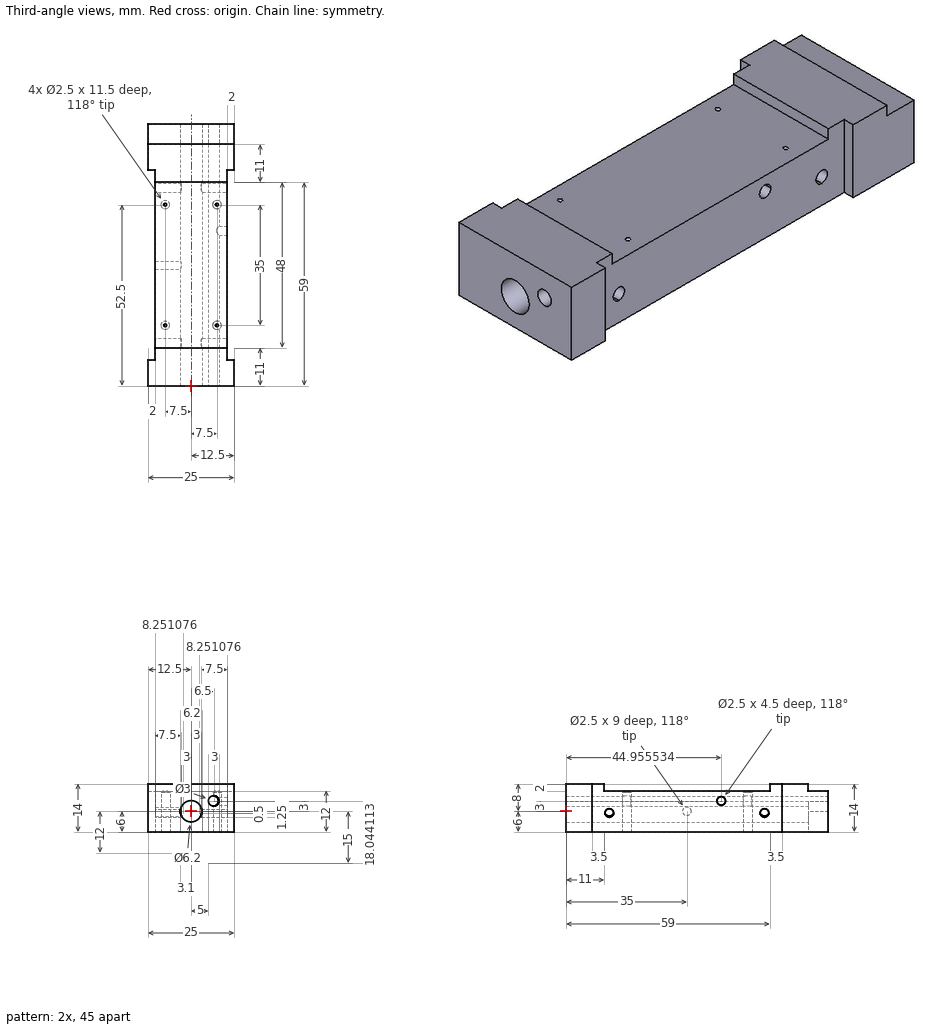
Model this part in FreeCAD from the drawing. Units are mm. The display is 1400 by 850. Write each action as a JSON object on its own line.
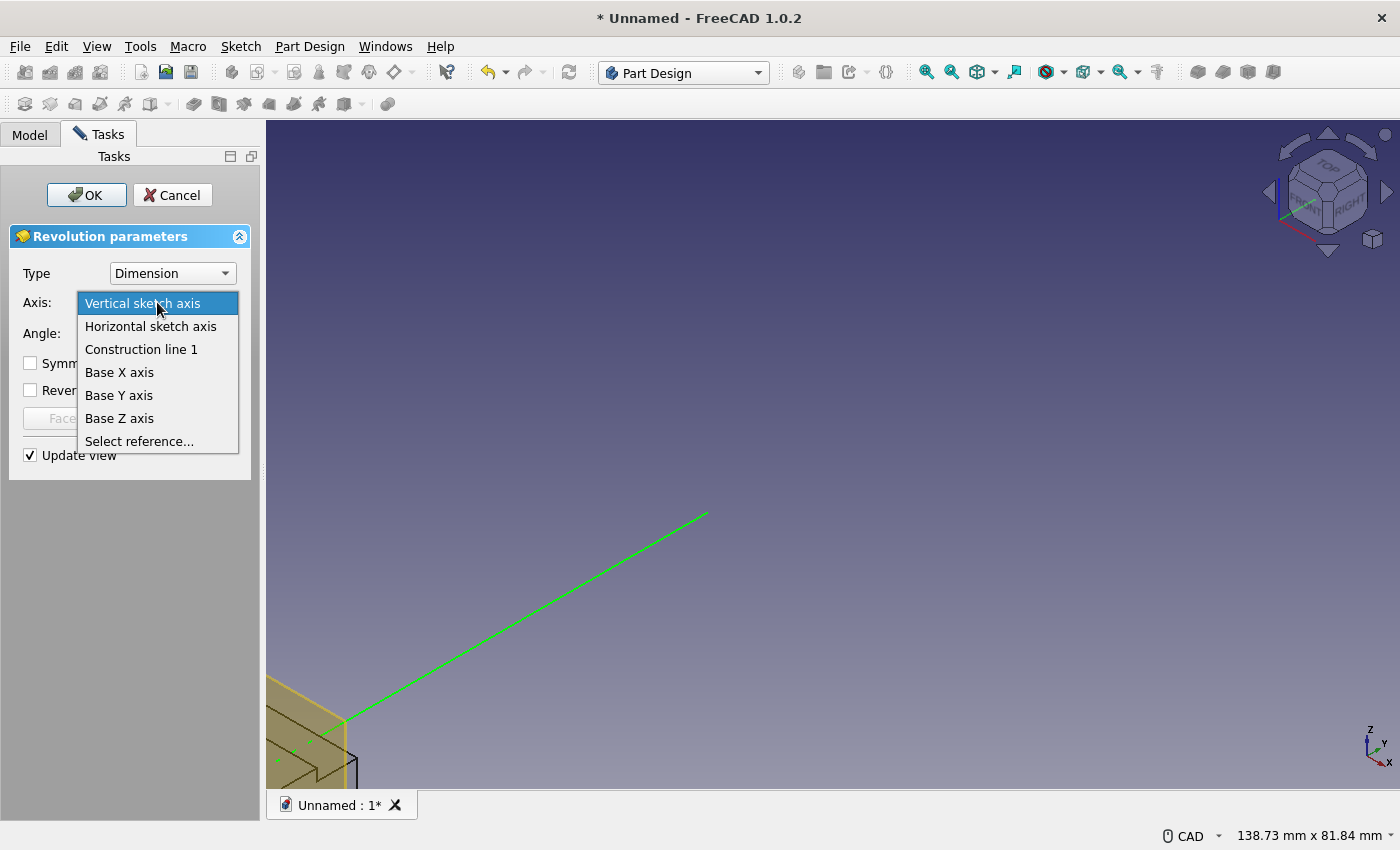
{"action": "left_click", "coordinate": [156, 350]}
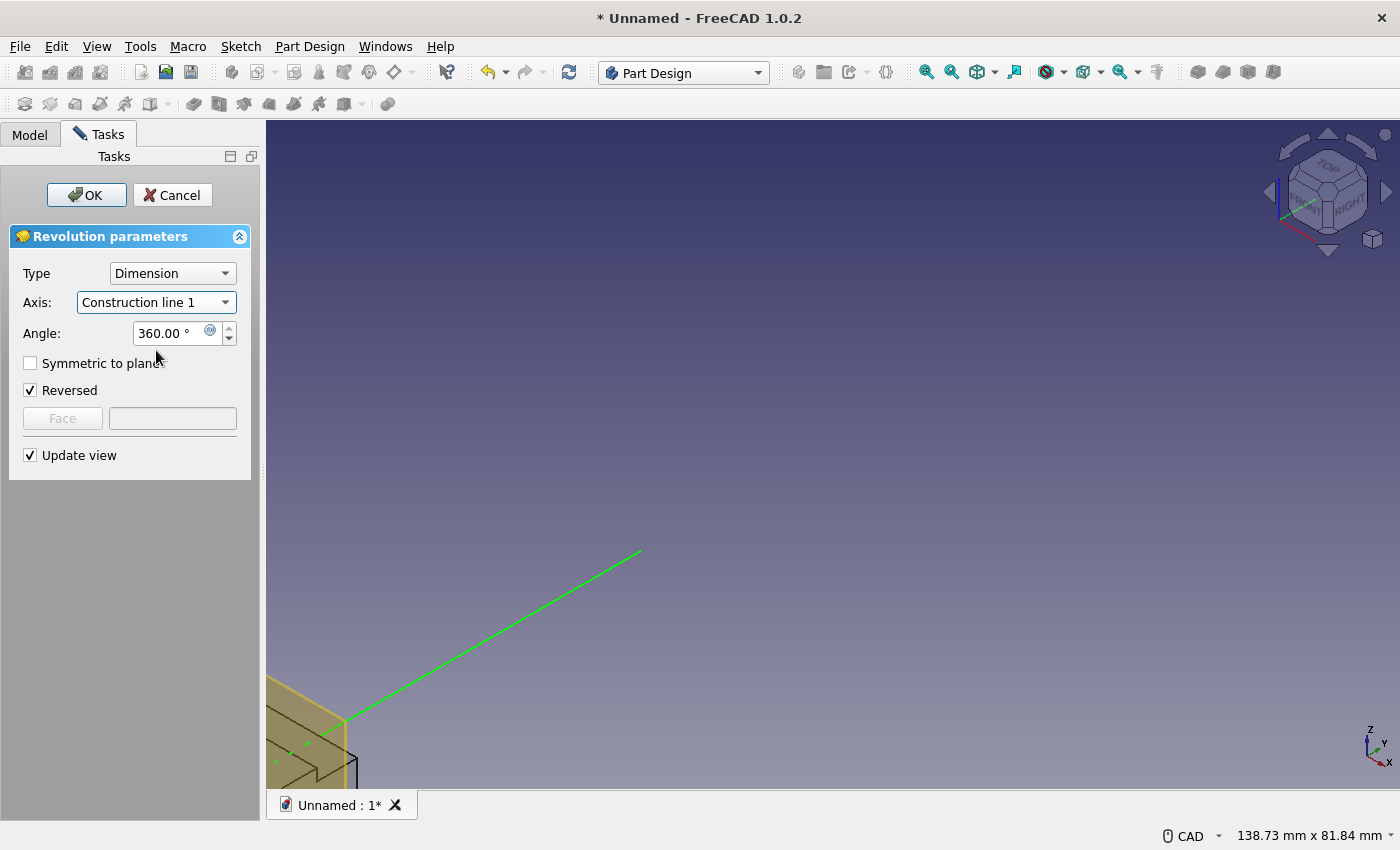
{"action": "left_click", "coordinate": [87, 195]}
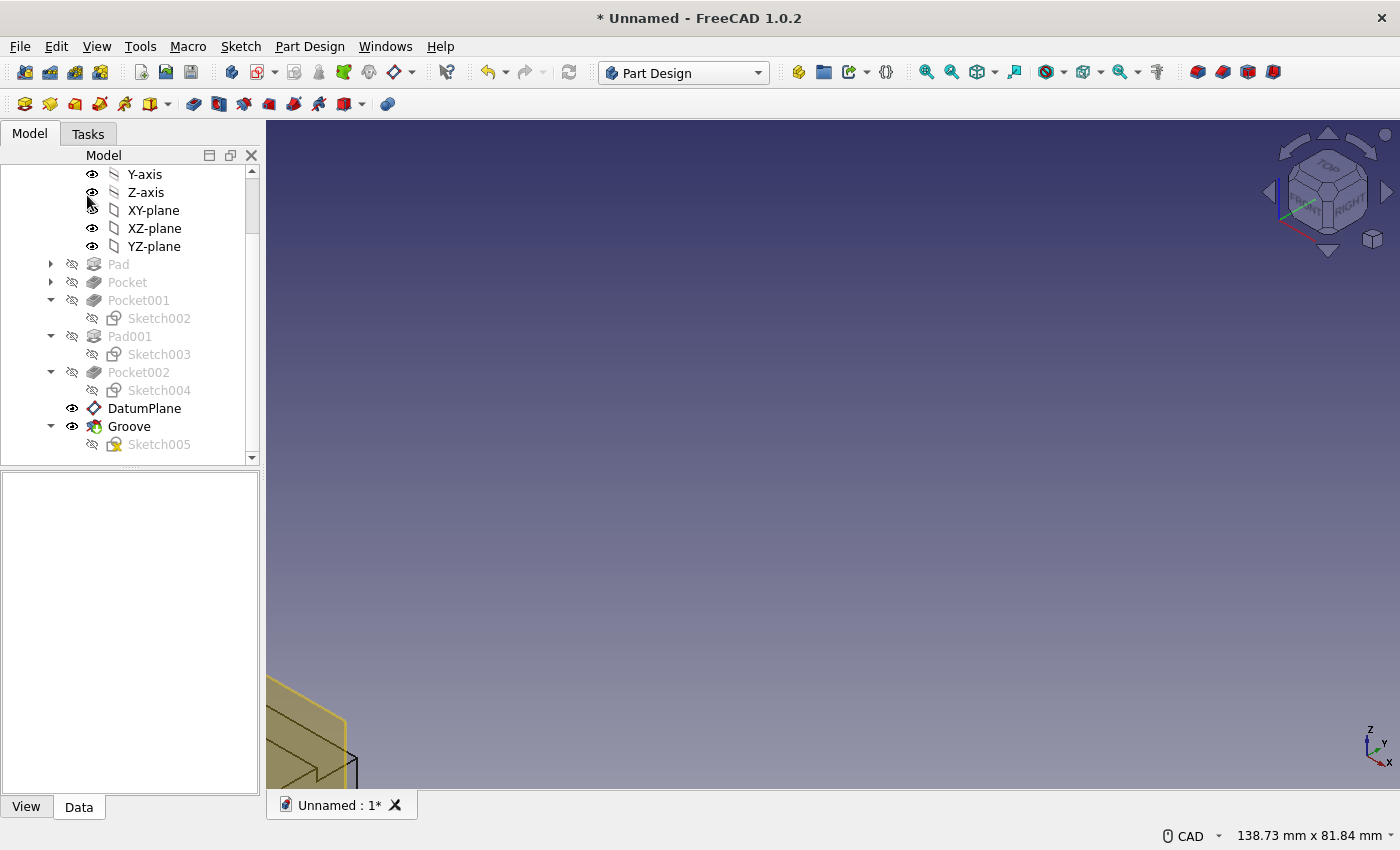
{"action": "left_click", "coordinate": [117, 408]}
{"action": "key", "text": "space"}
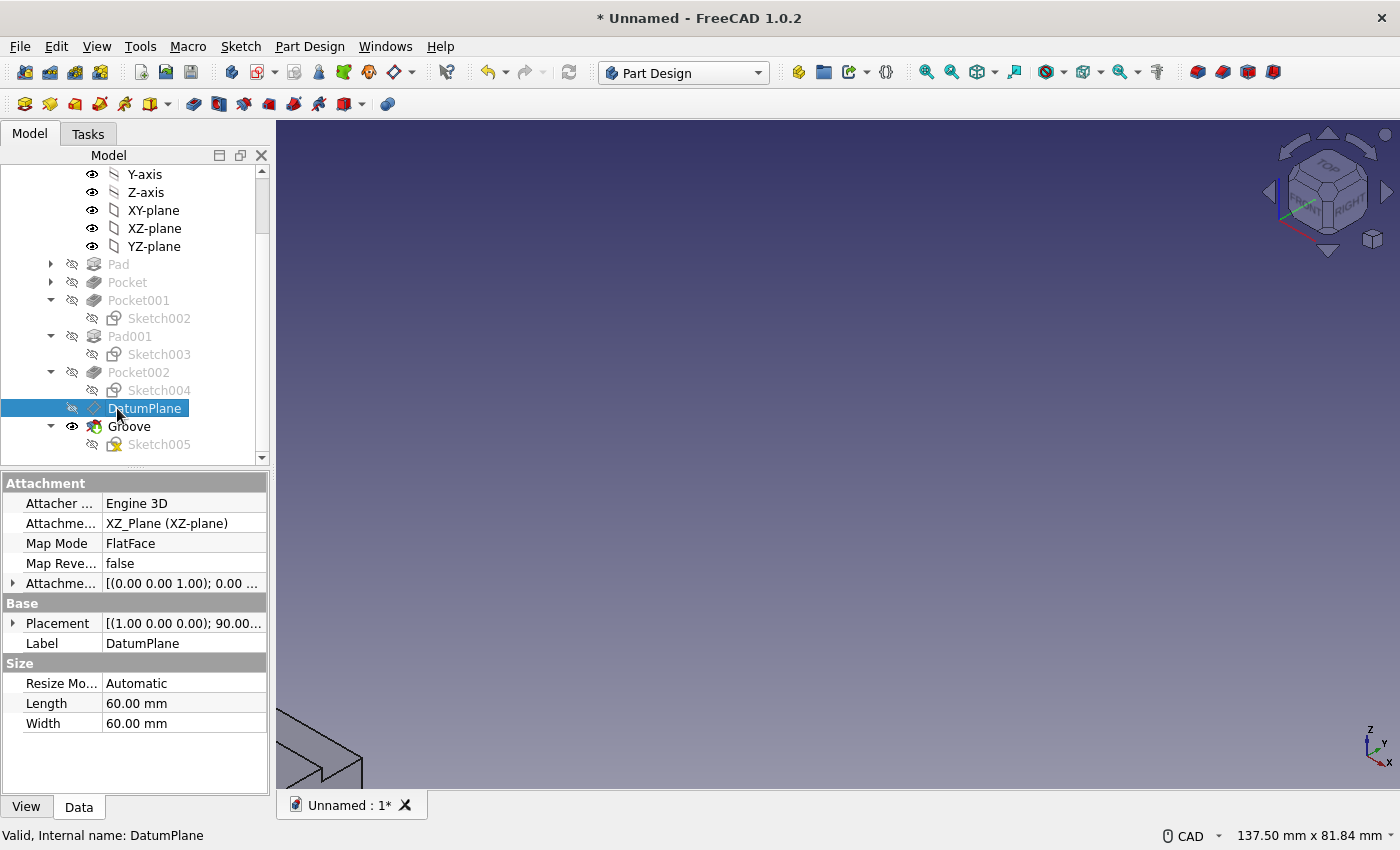
{"action": "left_click", "coordinate": [927, 72]}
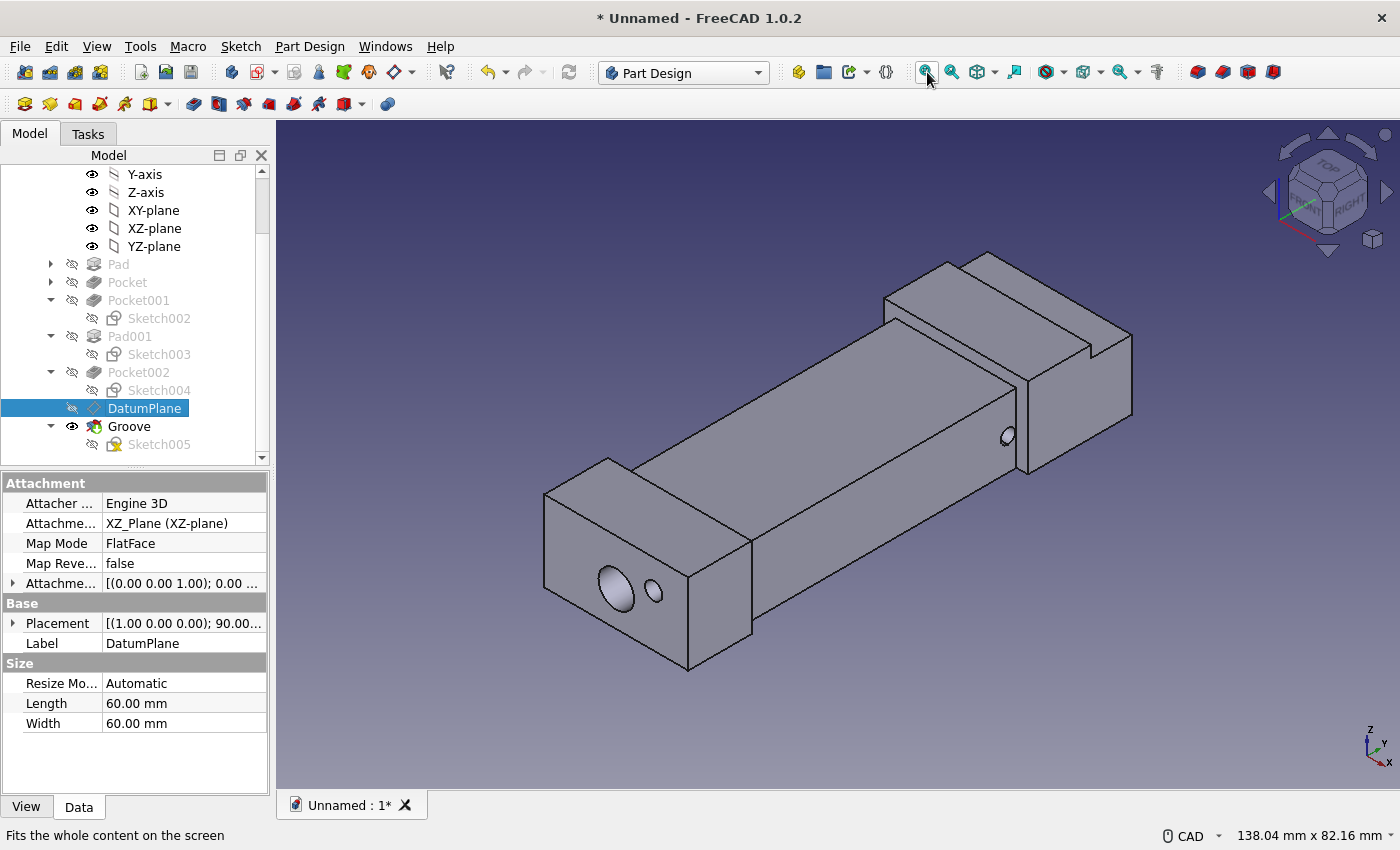
{"action": "left_click", "coordinate": [117, 426]}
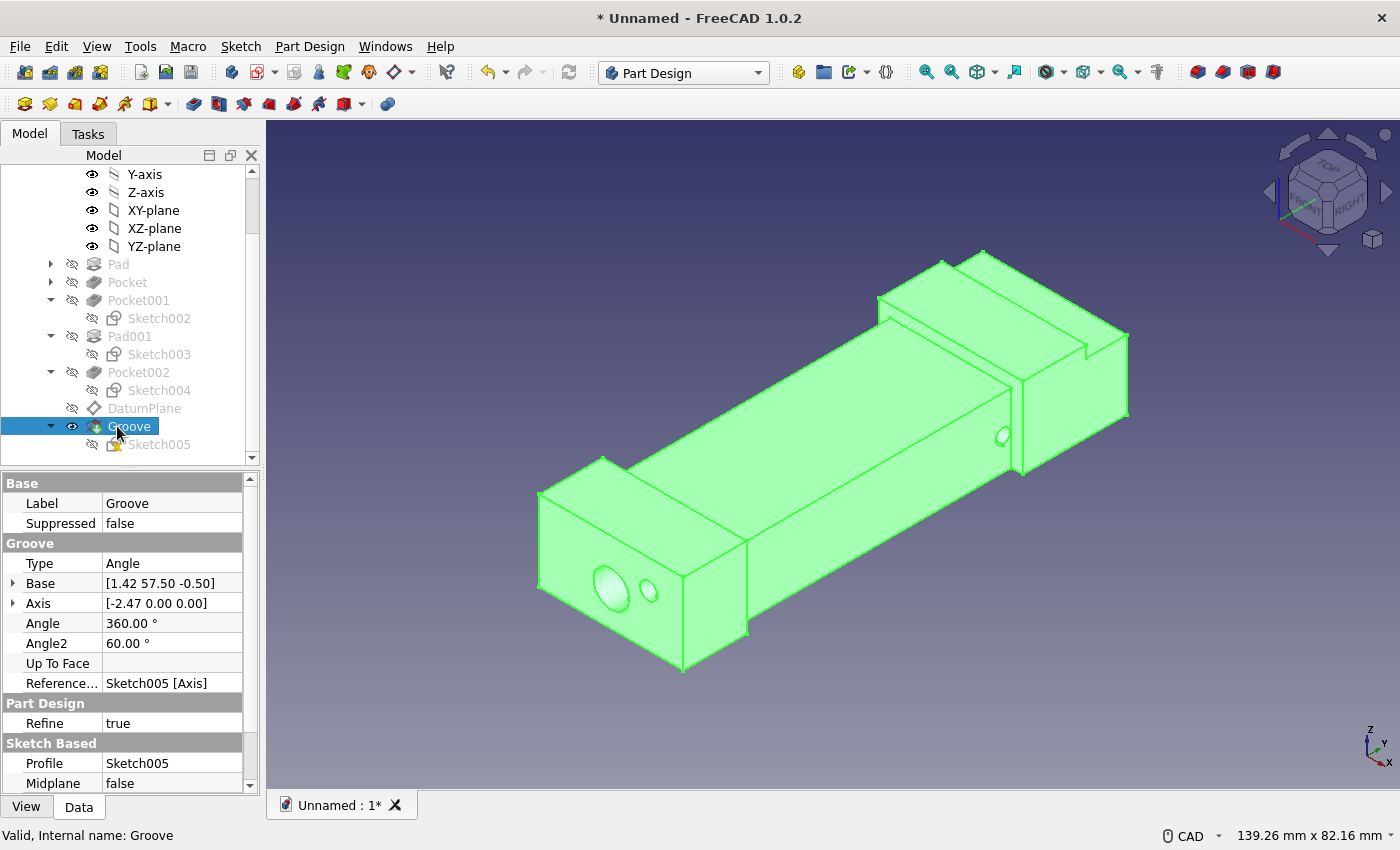
{"action": "left_click", "coordinate": [50, 72]}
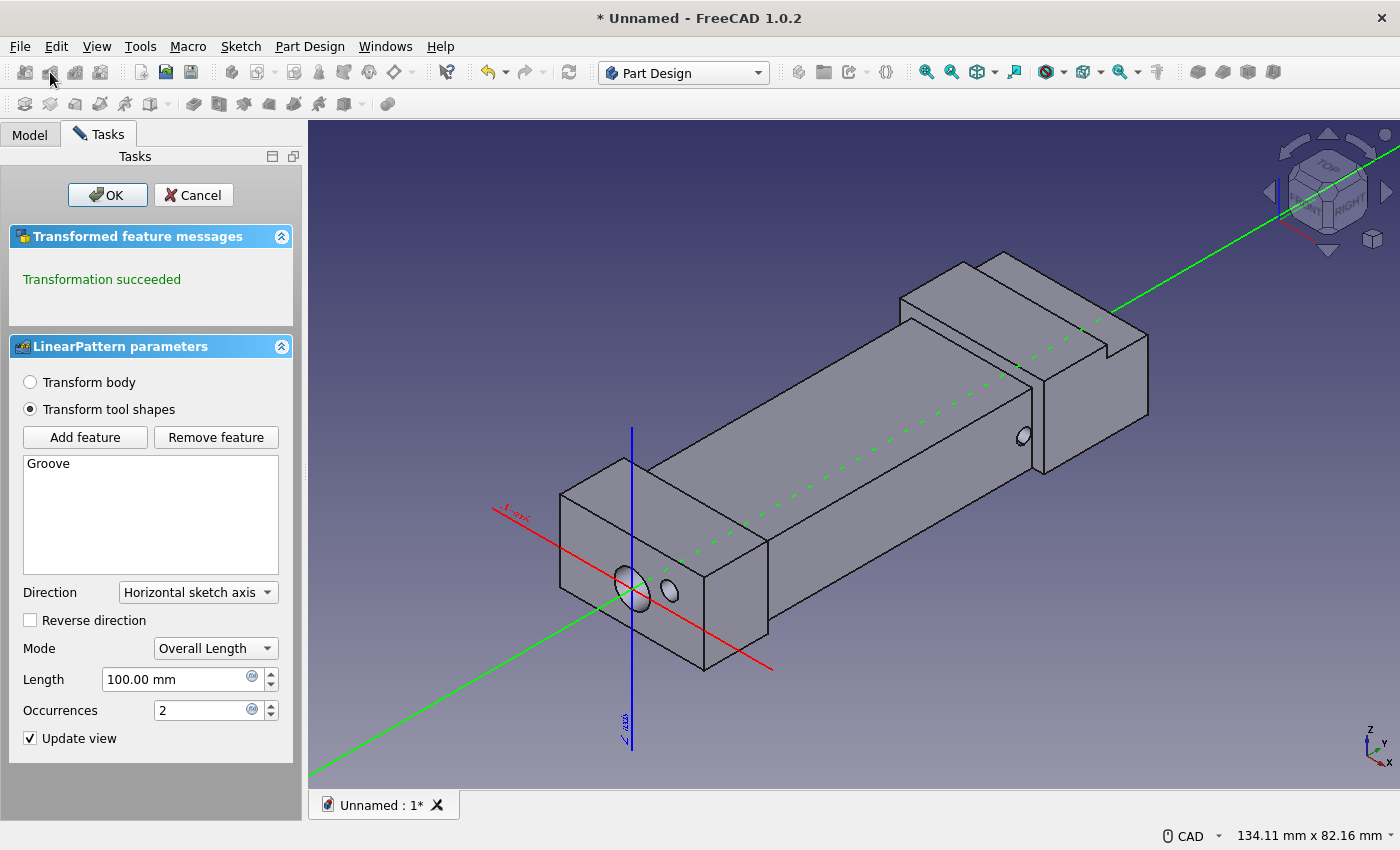
{"action": "left_click", "coordinate": [199, 592]}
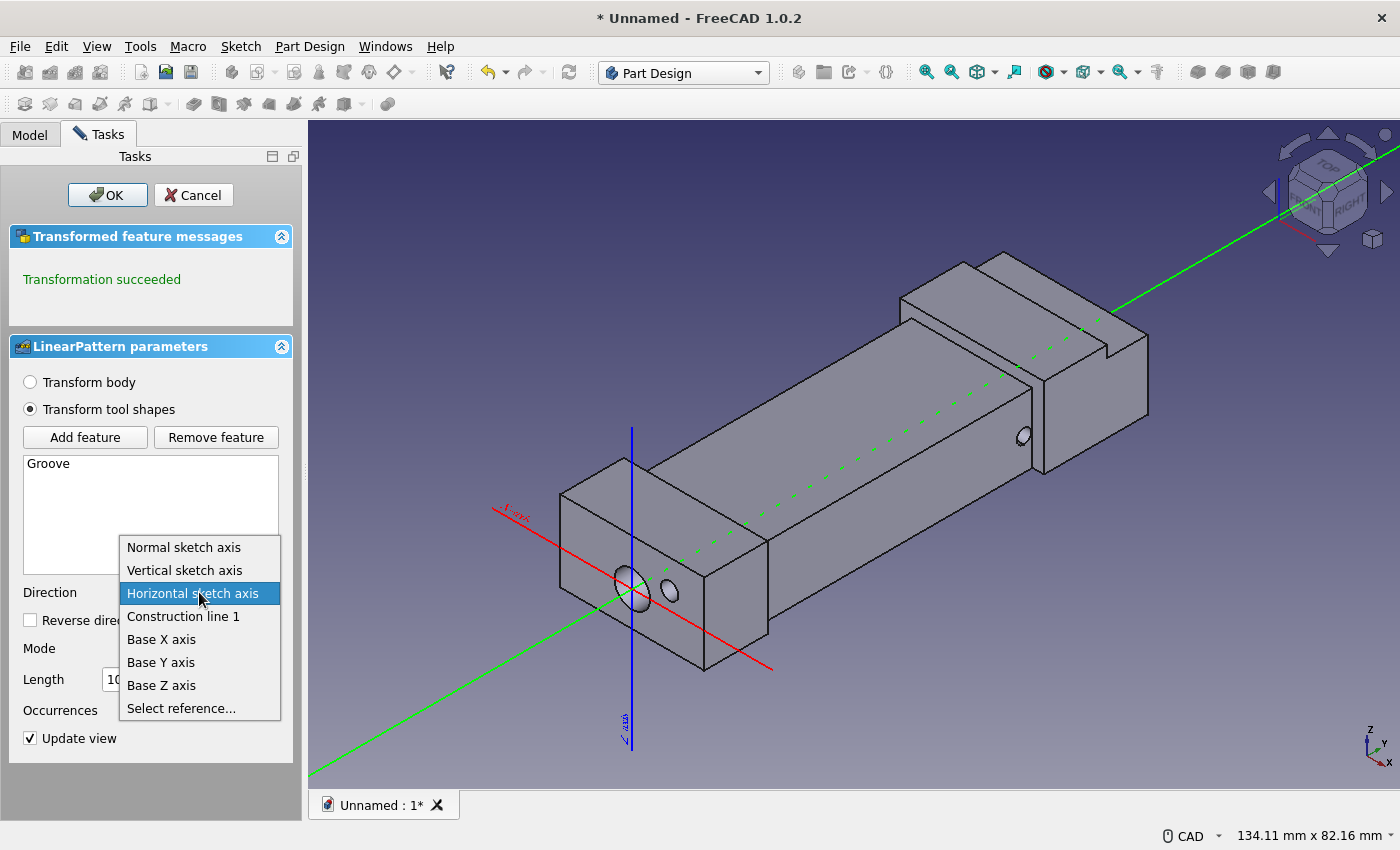
{"action": "left_click", "coordinate": [198, 662]}